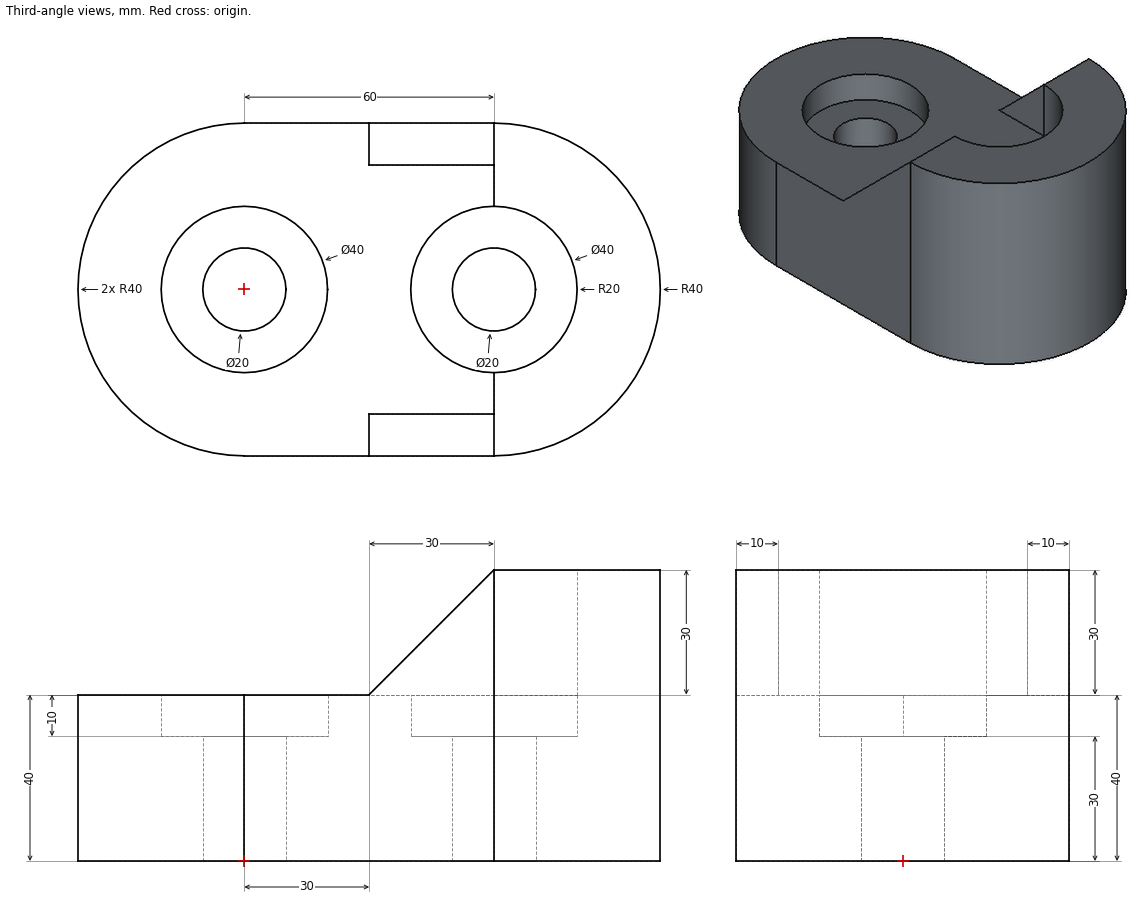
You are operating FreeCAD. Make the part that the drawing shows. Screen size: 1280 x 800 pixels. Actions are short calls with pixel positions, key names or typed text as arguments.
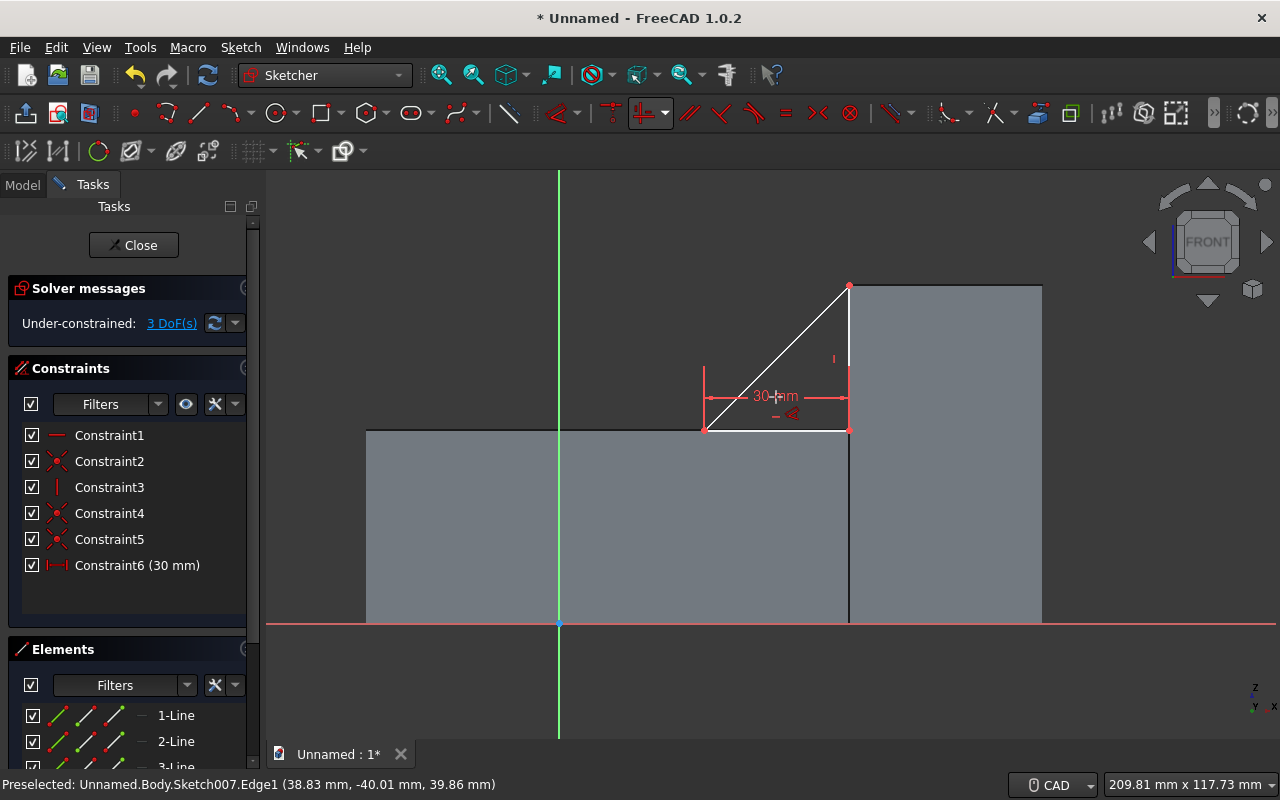
click(849, 387)
click(883, 358)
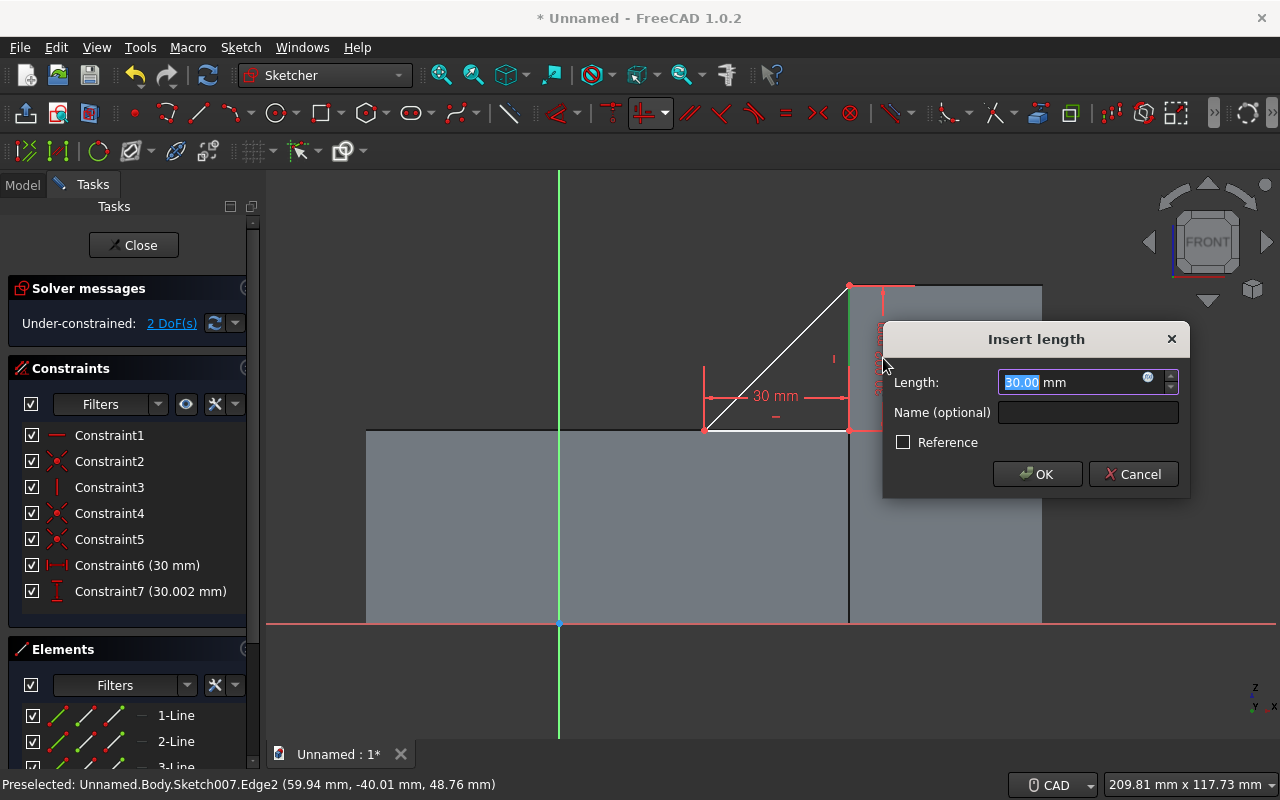
text(30)
key(Return)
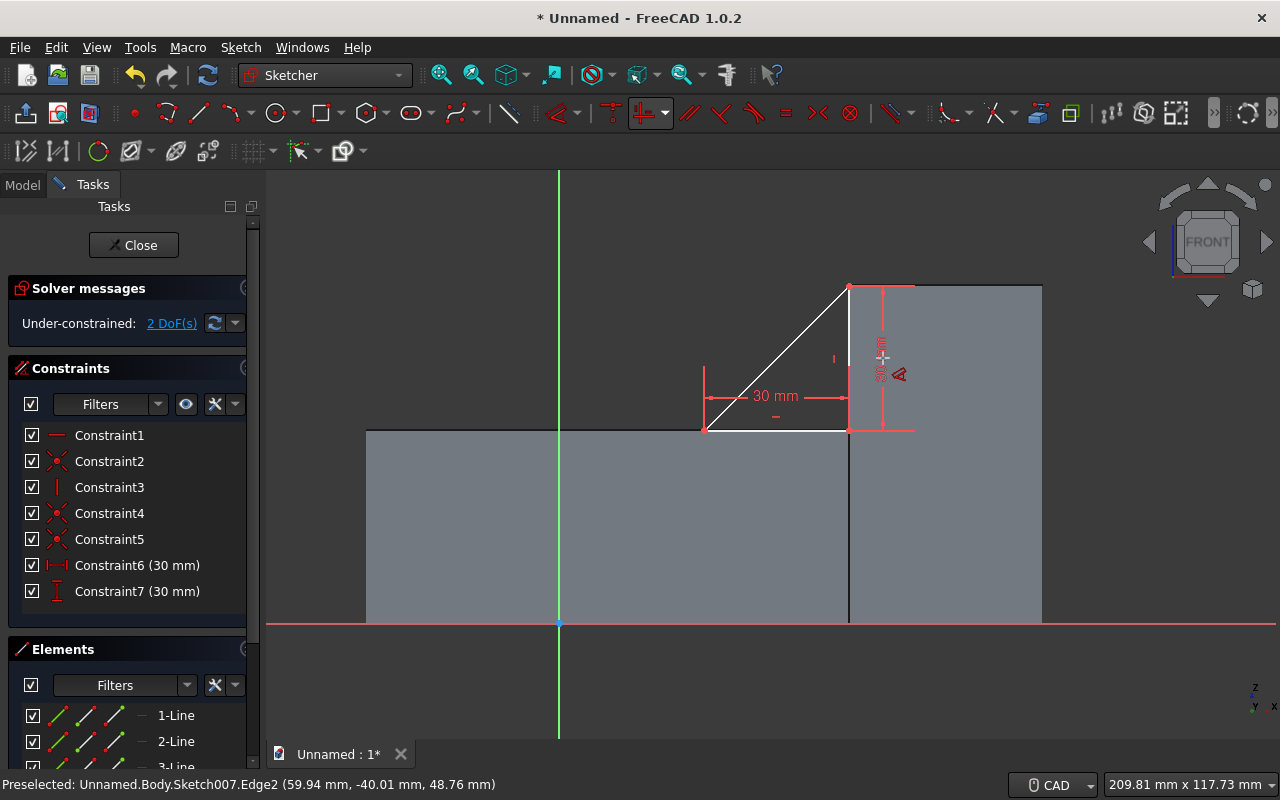
click(704, 431)
click(632, 658)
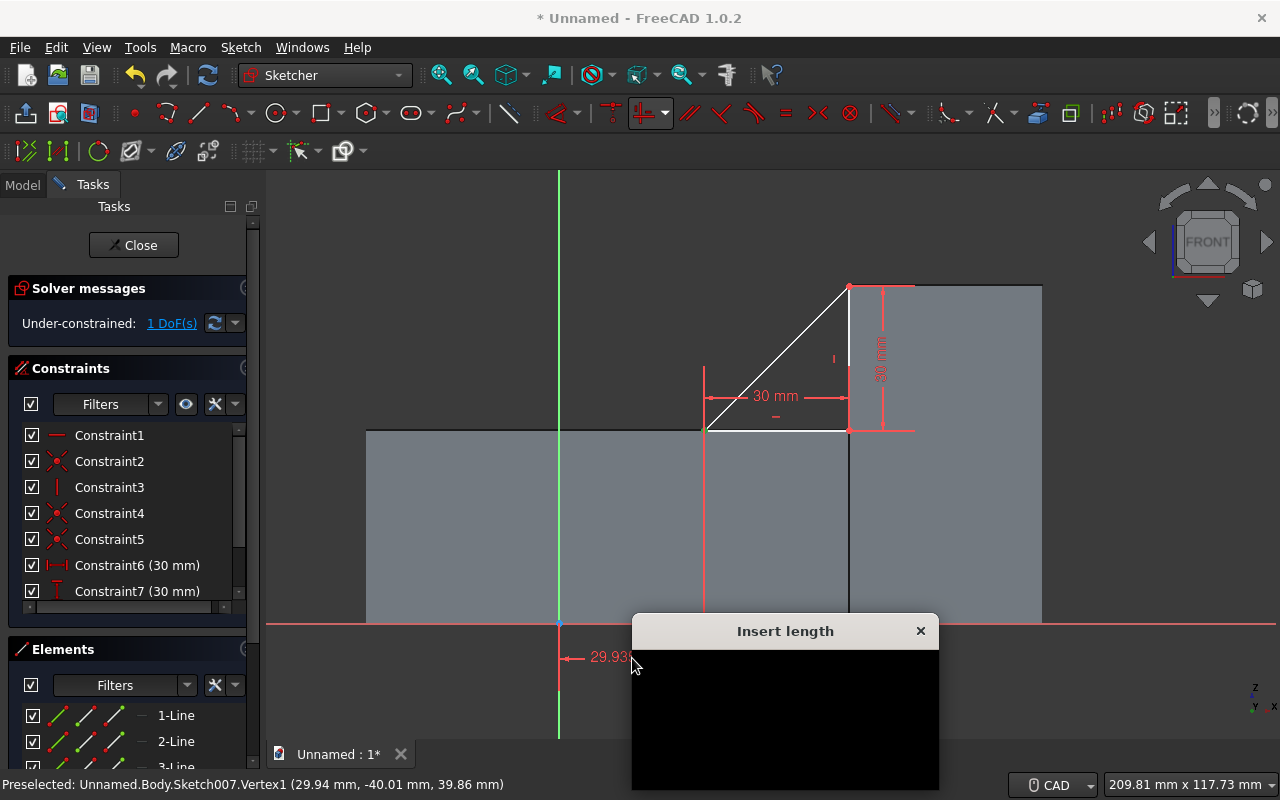
text(30)
key(Return)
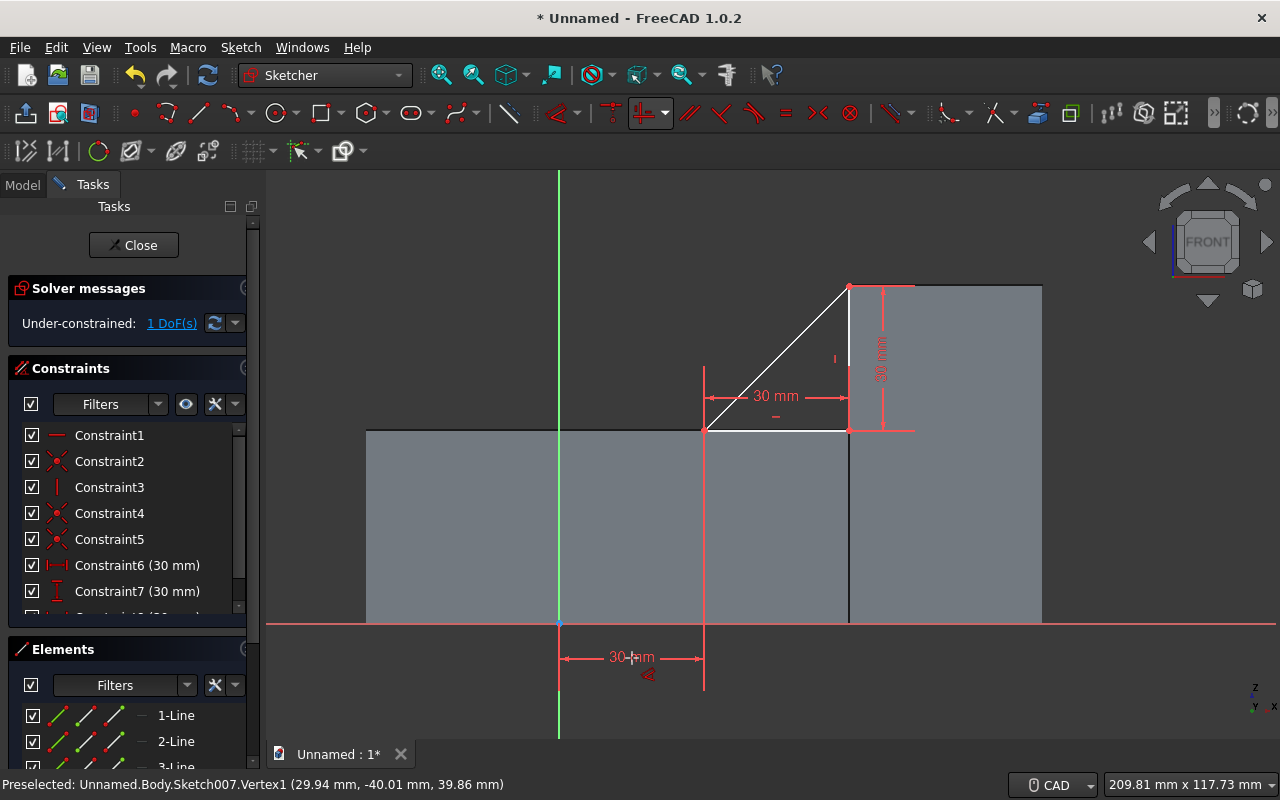
click(704, 431)
click(525, 527)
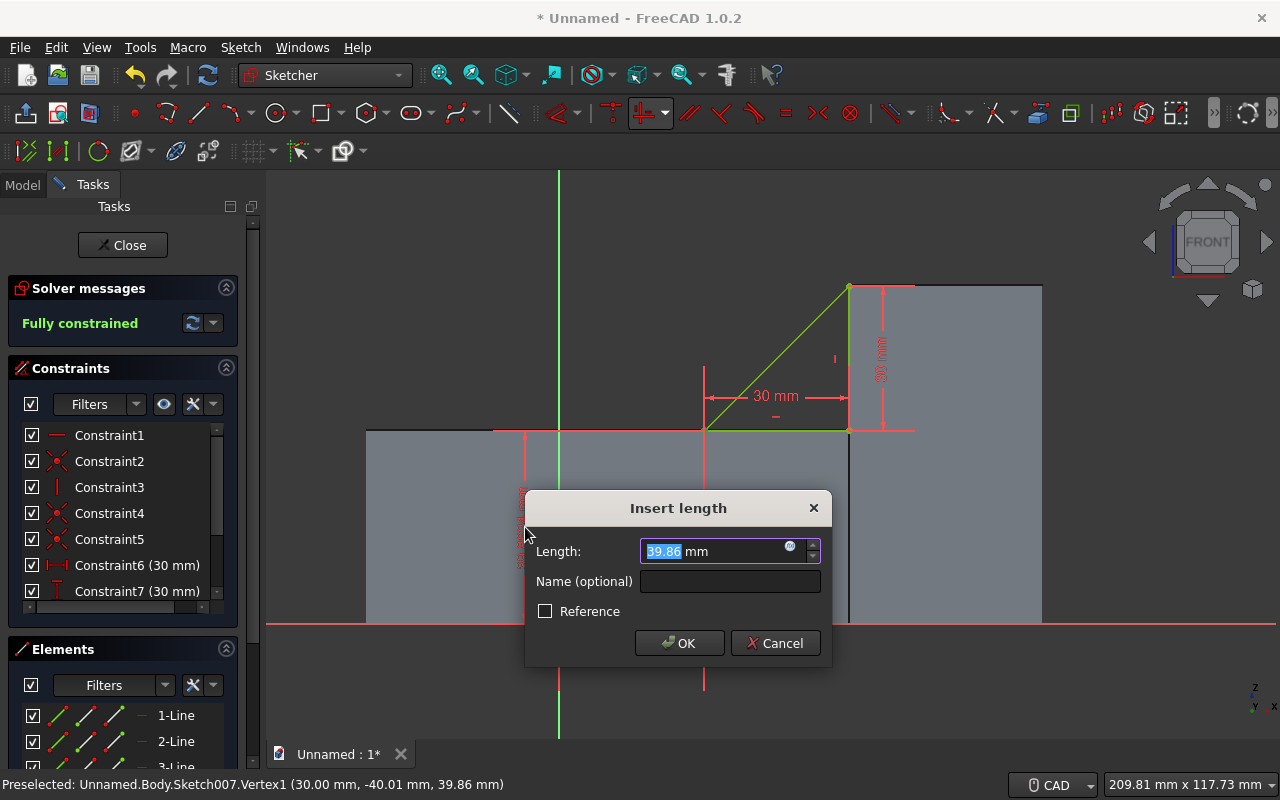
text(40)
key(Return)
key(Escape)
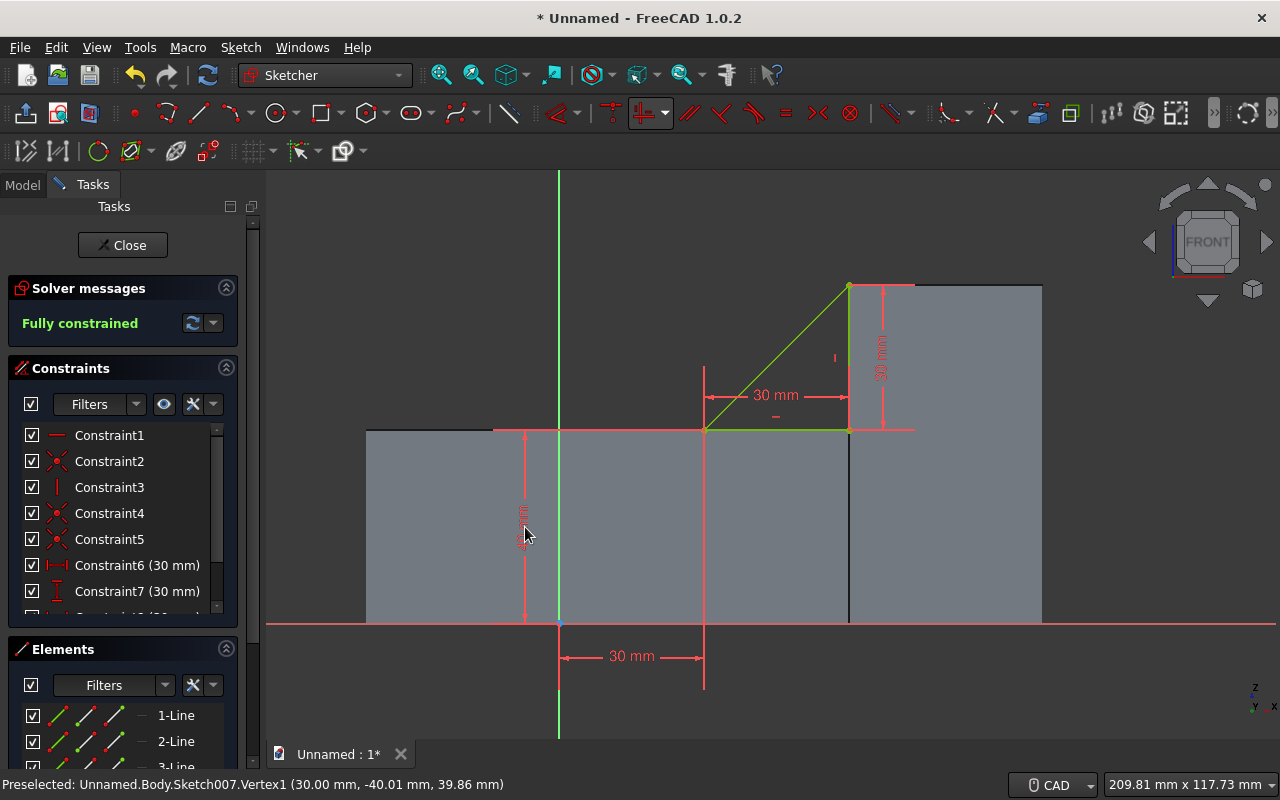
click(123, 245)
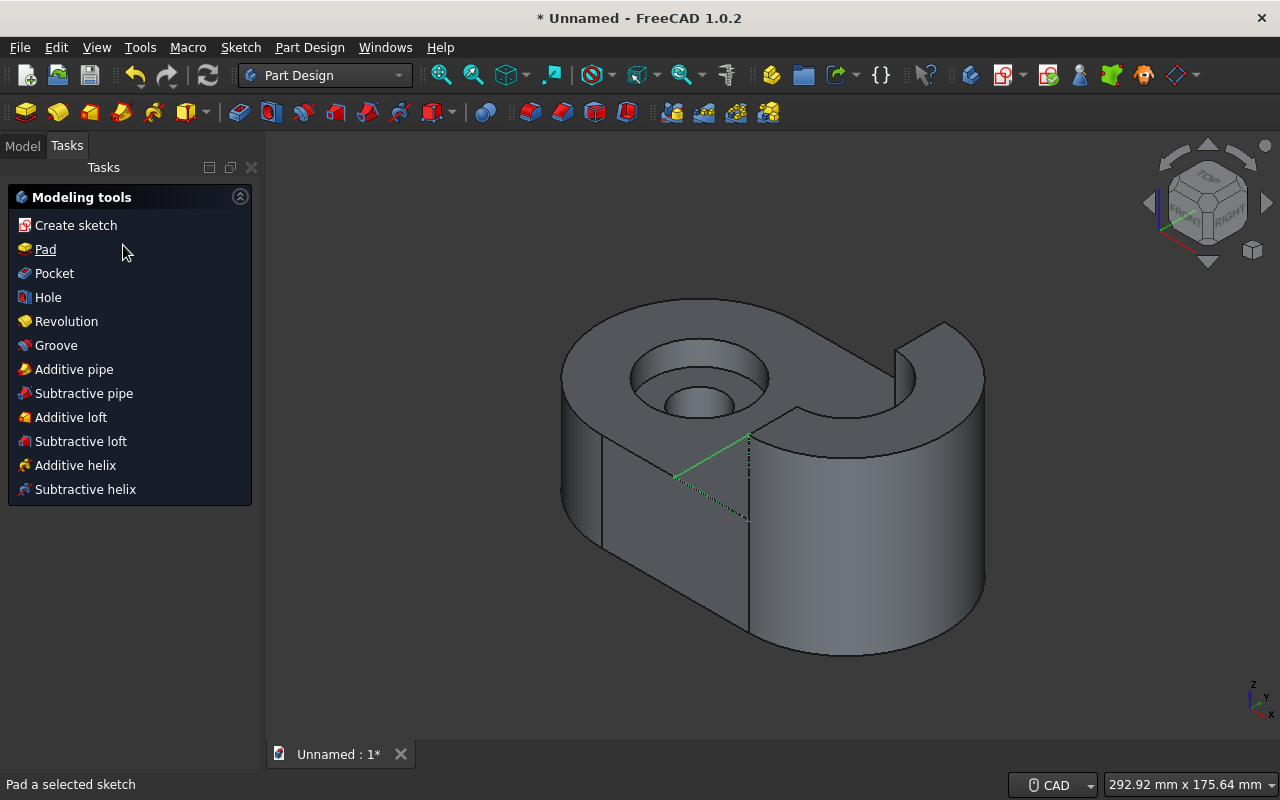
click(26, 112)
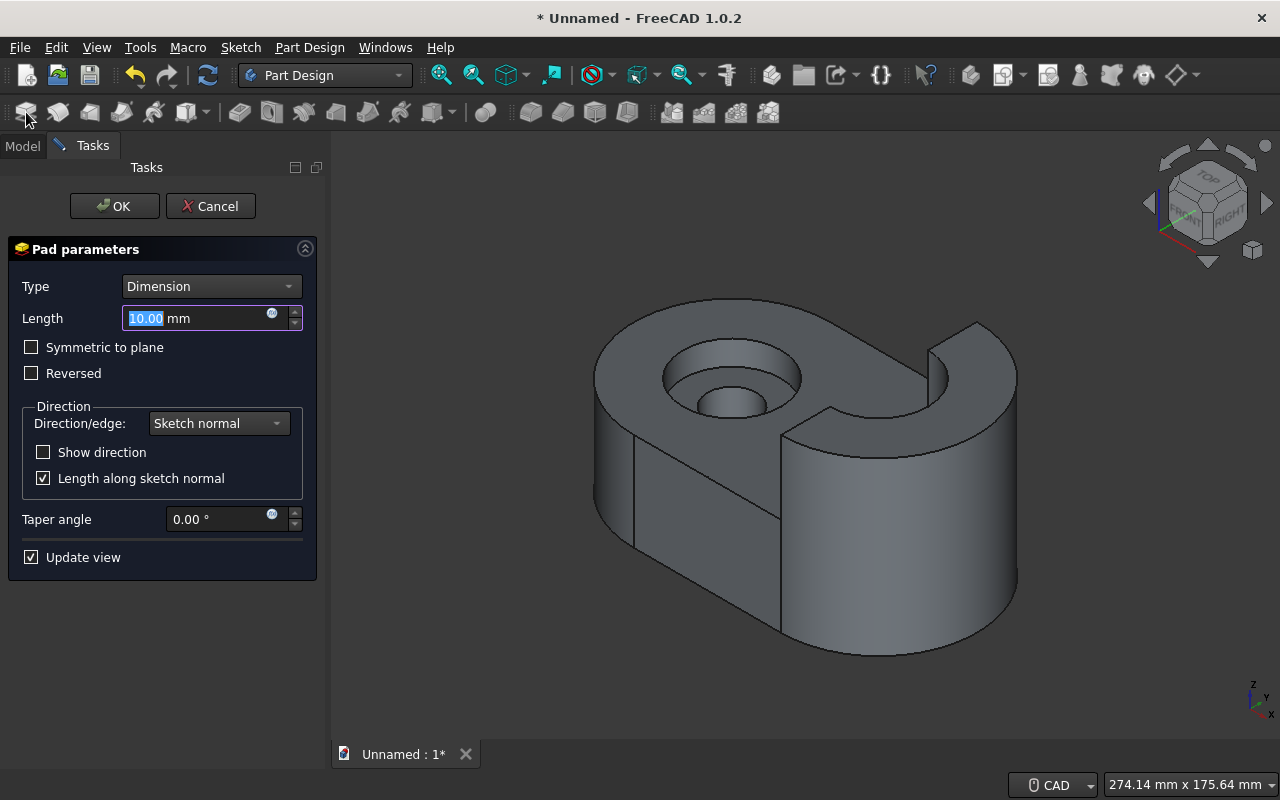
text(10)
key(Tab)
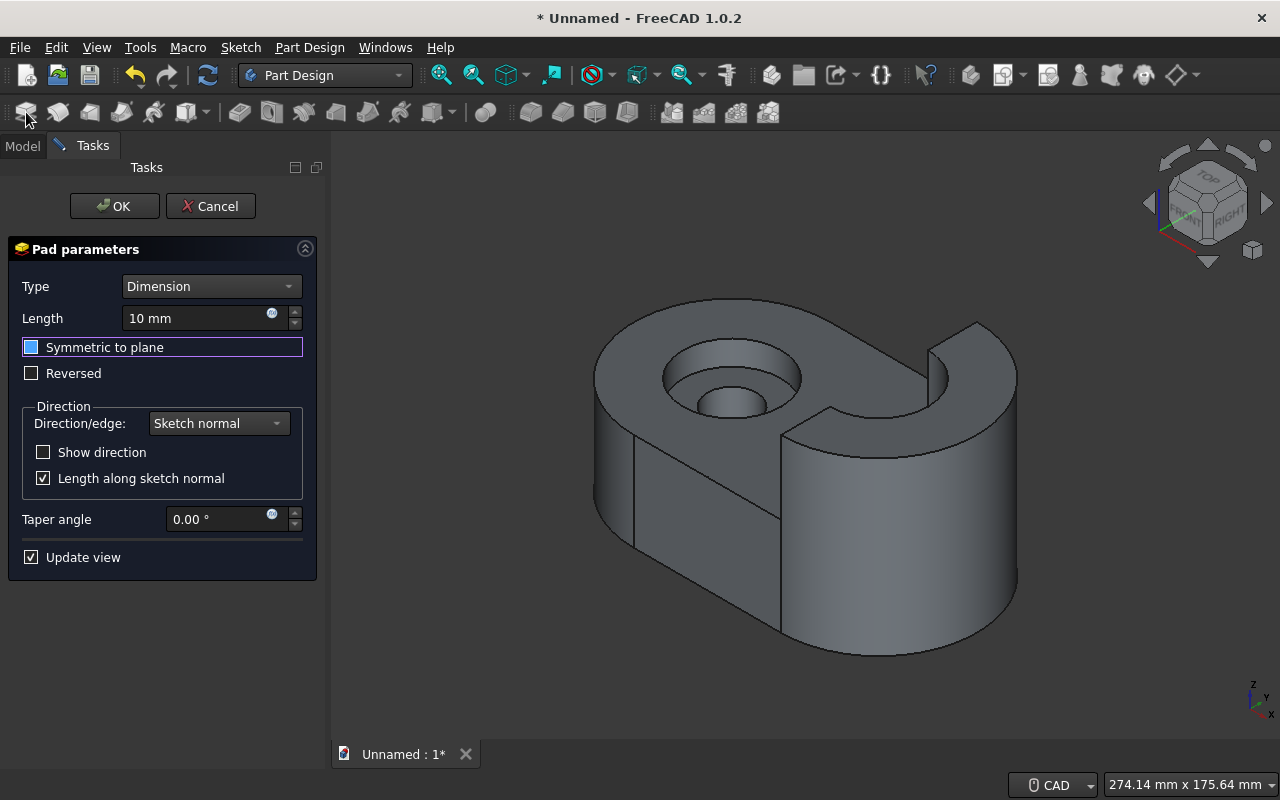
click(30, 373)